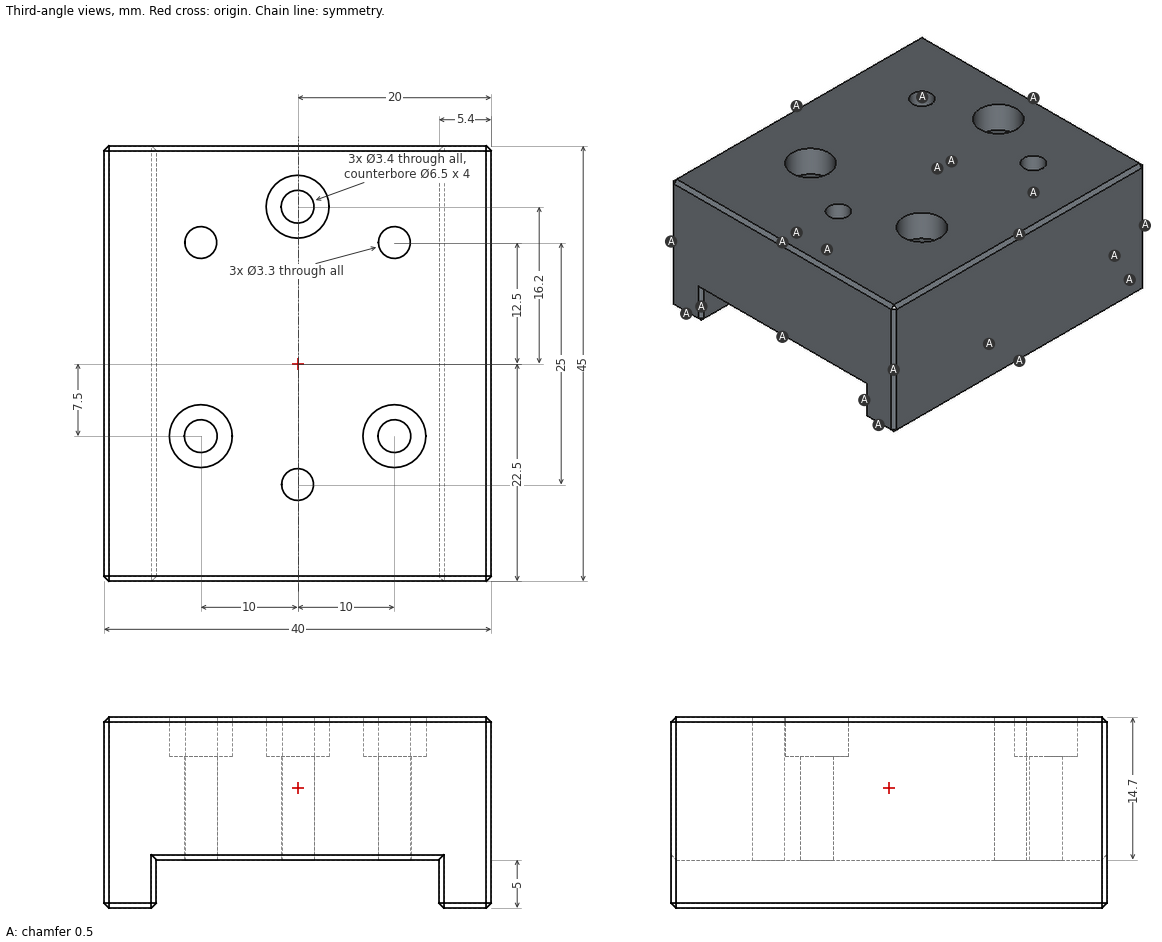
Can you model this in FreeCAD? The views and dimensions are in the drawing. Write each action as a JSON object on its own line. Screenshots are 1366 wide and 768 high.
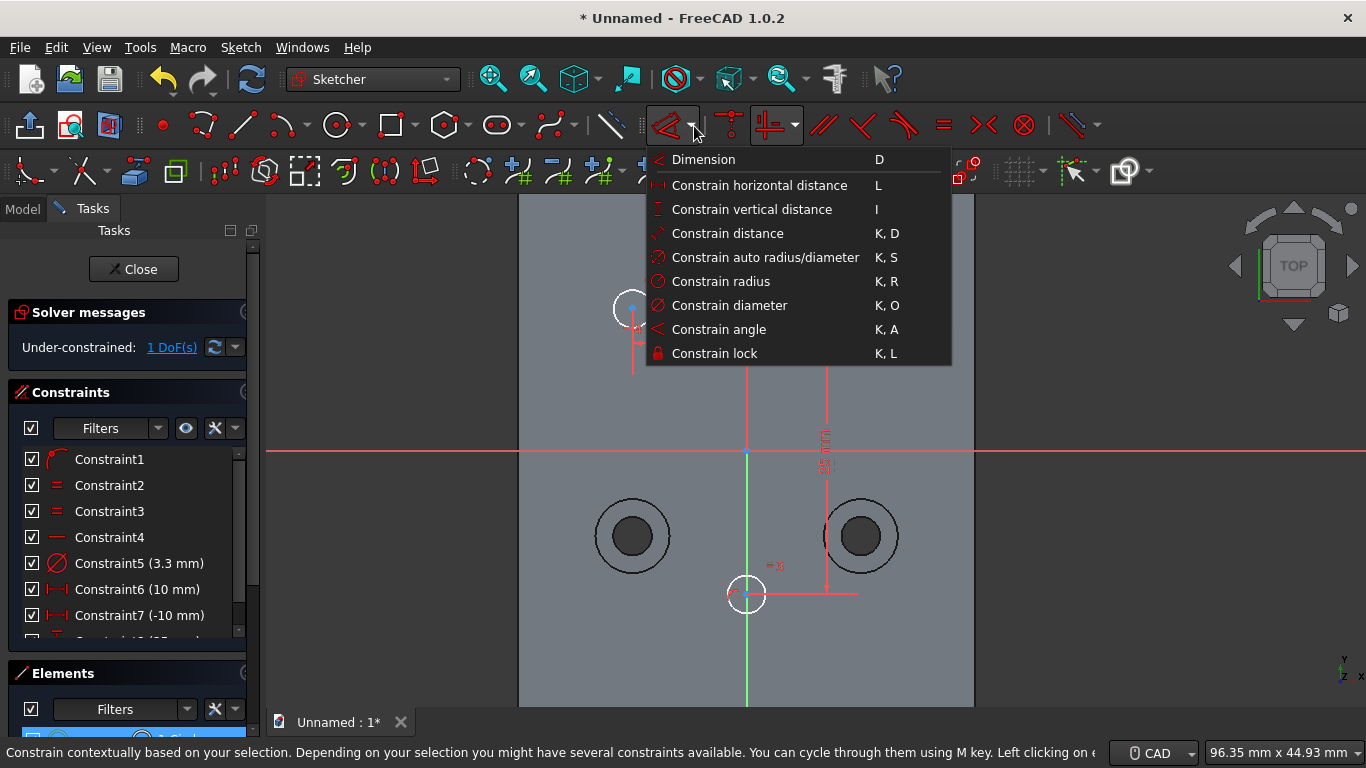
{"action": "left_click", "coordinate": [799, 209]}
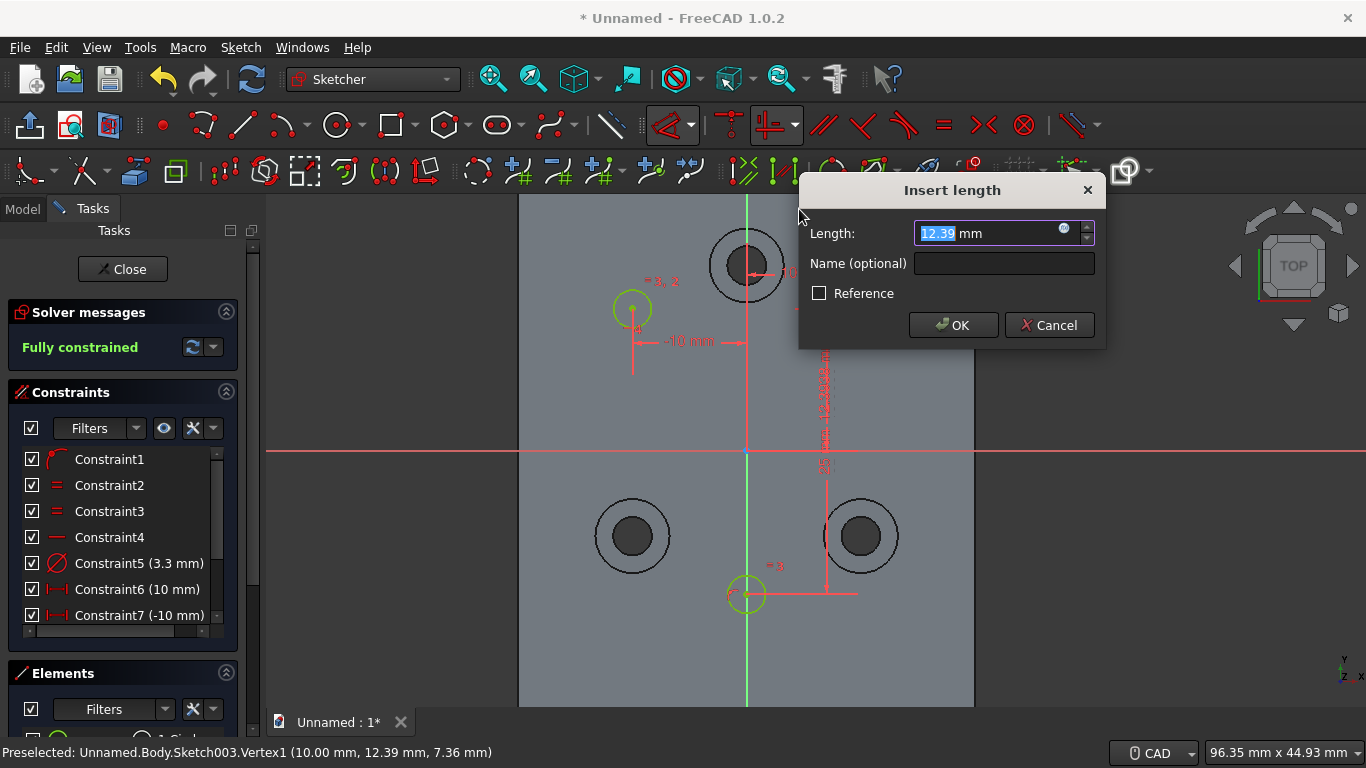
{"action": "type", "text": "12.5"}
{"action": "key", "text": "Return"}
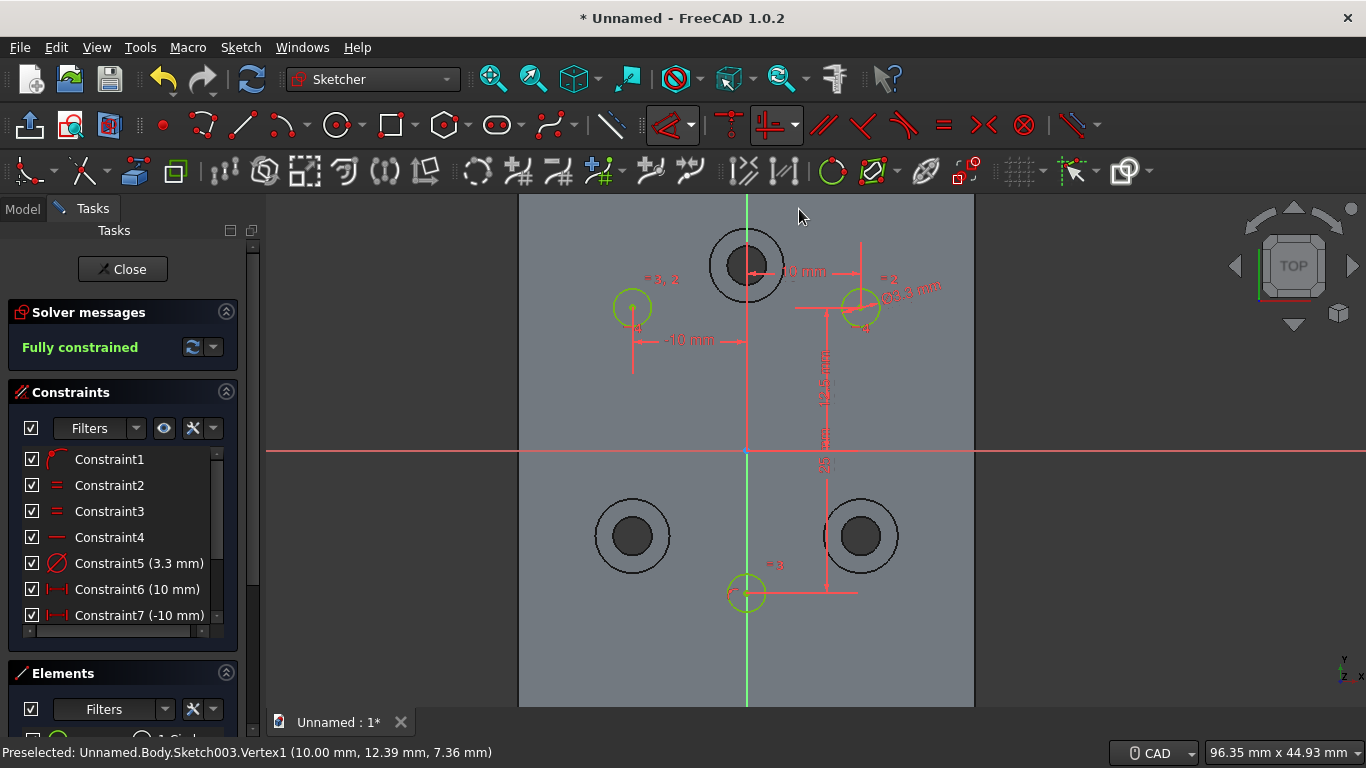
{"action": "left_click", "coordinate": [123, 269]}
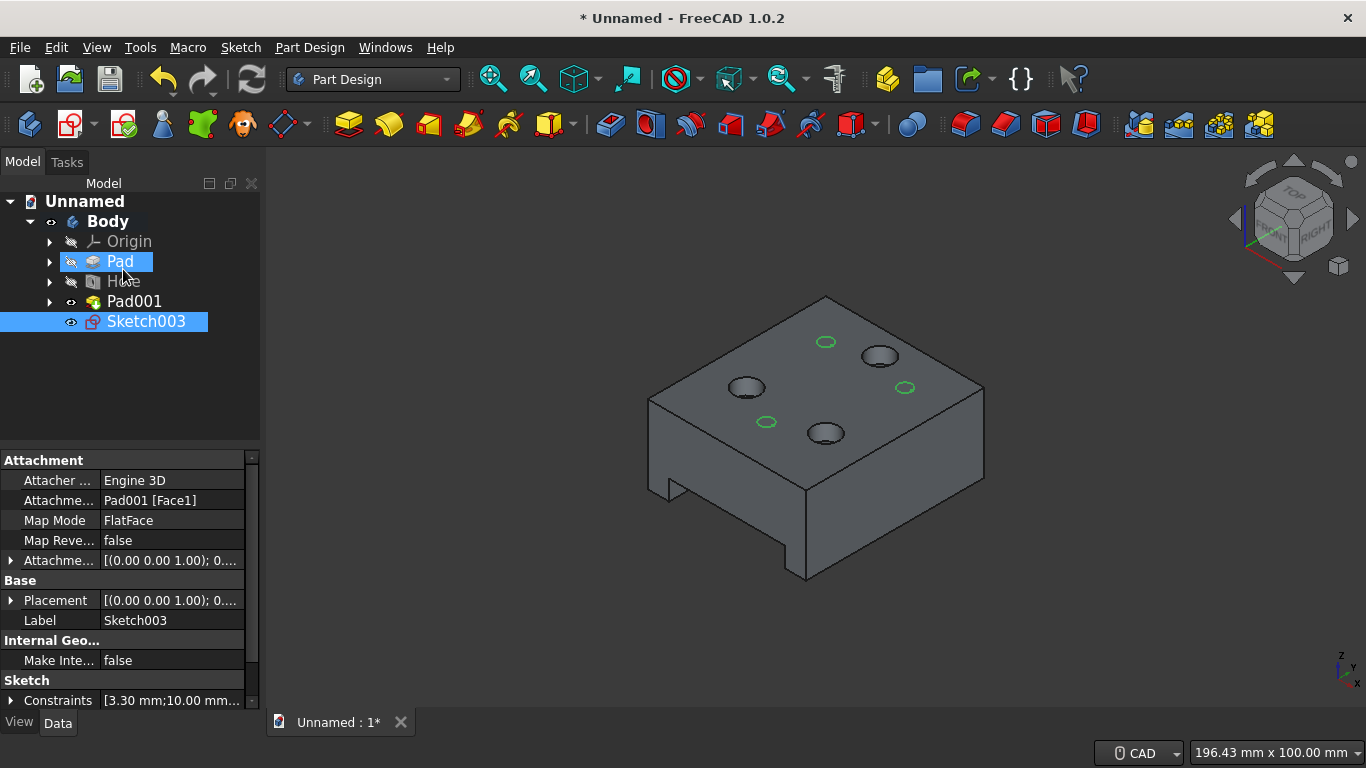
{"action": "left_click", "coordinate": [652, 124]}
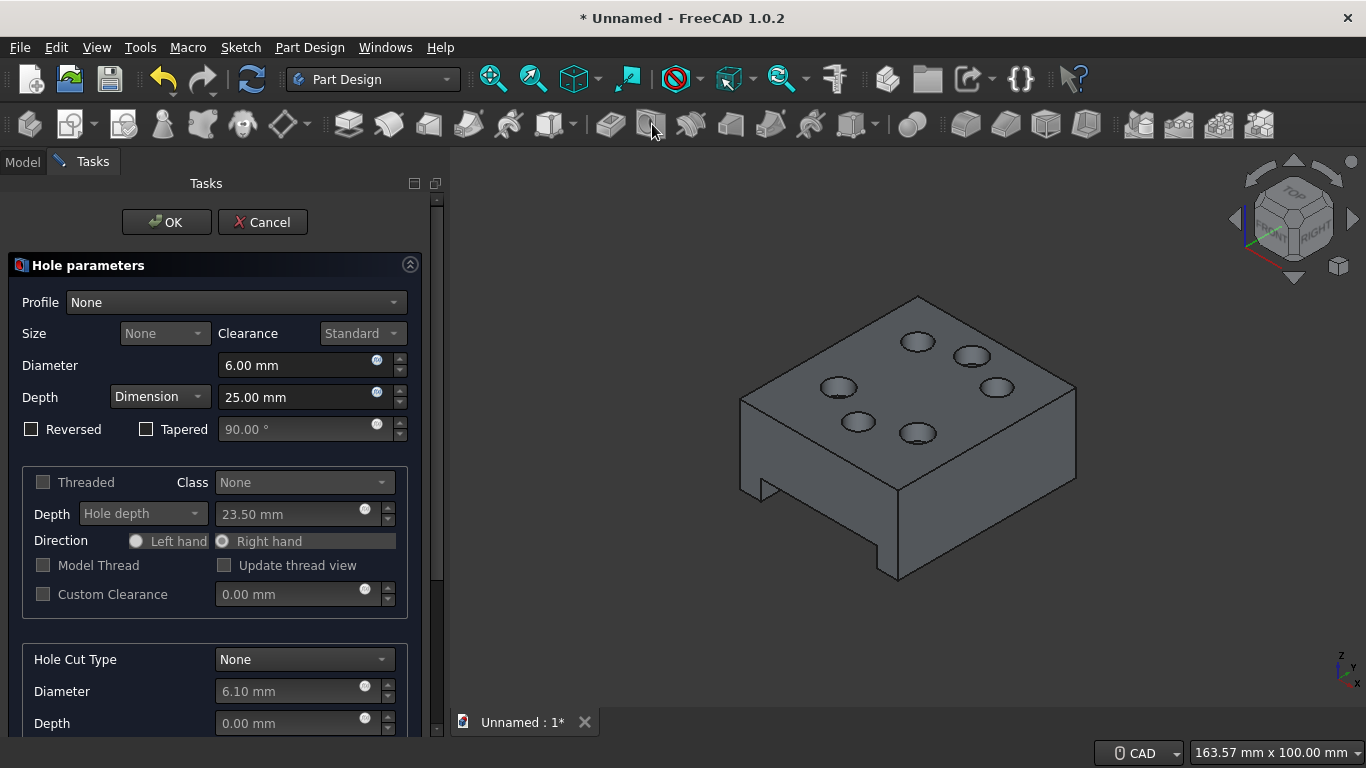
{"action": "triple_click", "coordinate": [305, 365]}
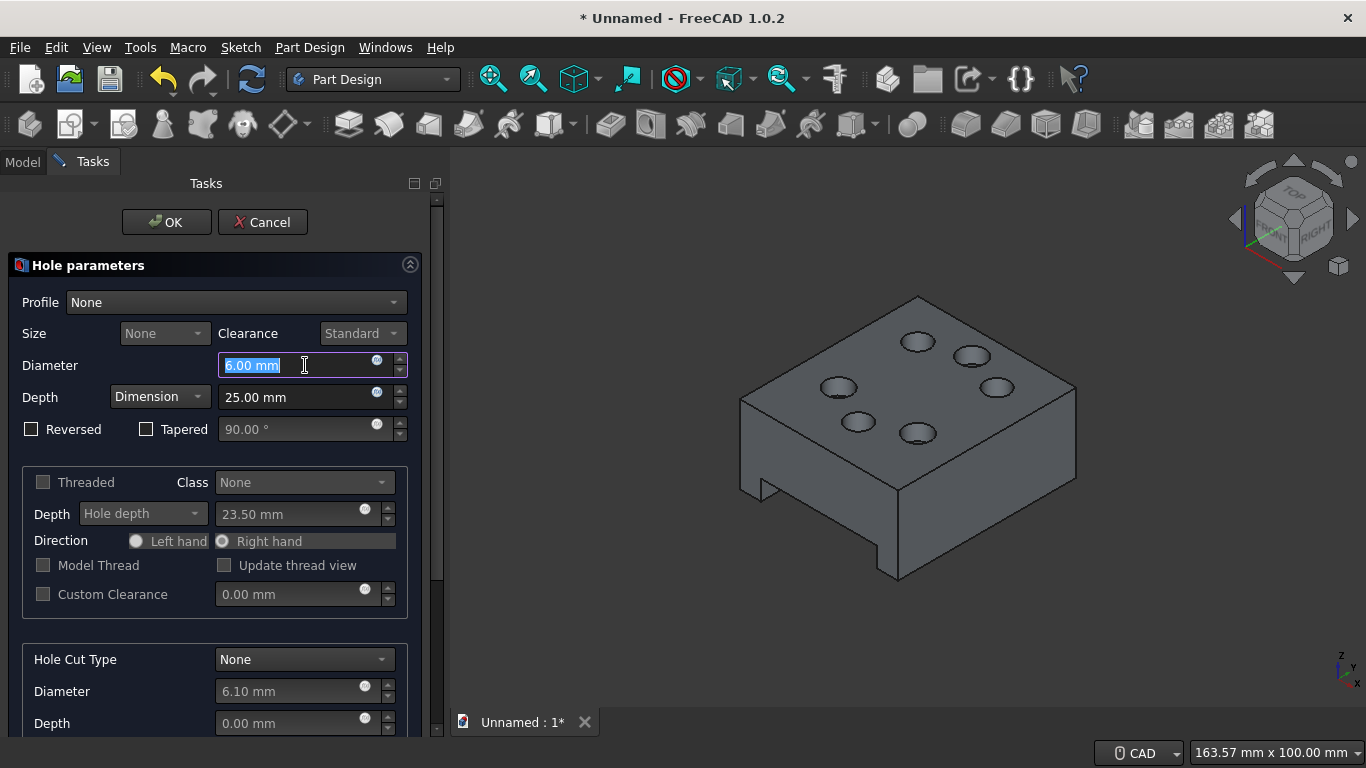
{"action": "type", "text": "3.3"}
{"action": "key", "text": "Tab"}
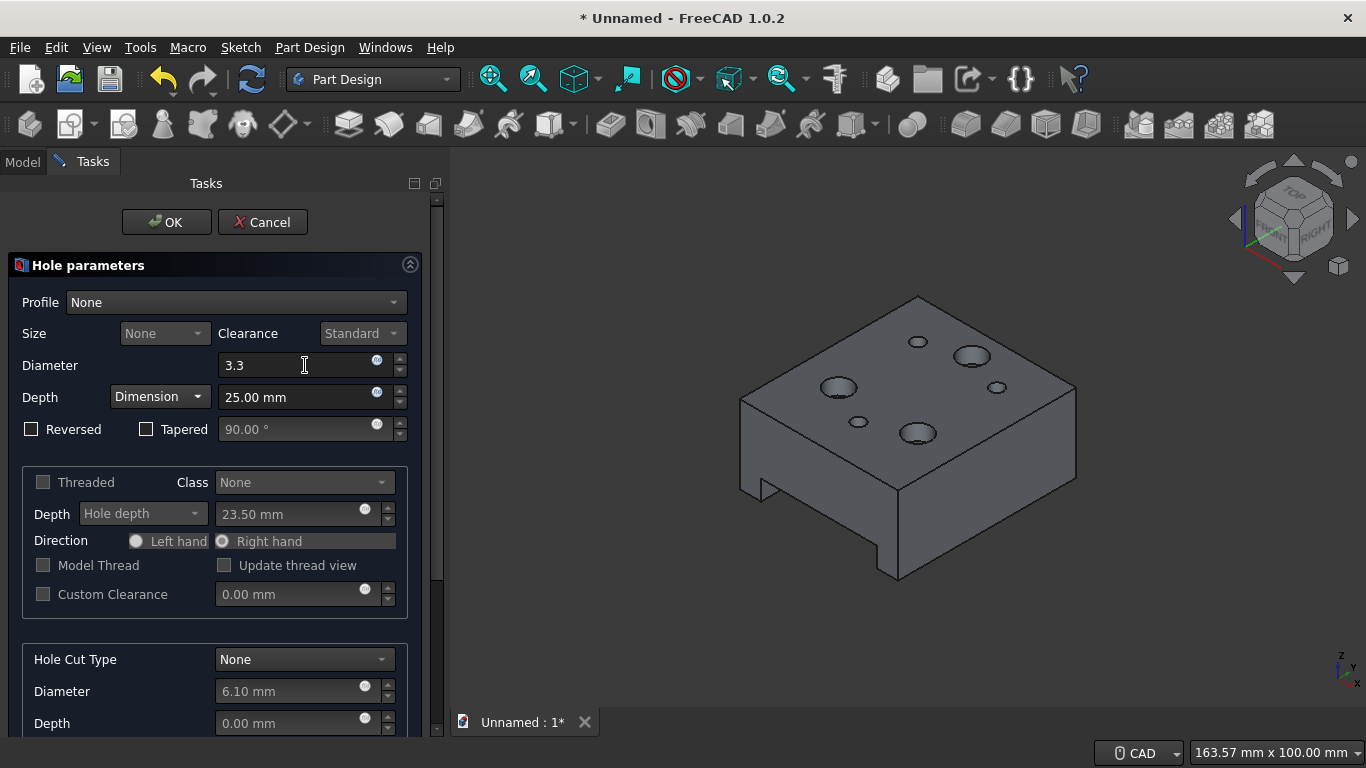
{"action": "left_click", "coordinate": [161, 396]}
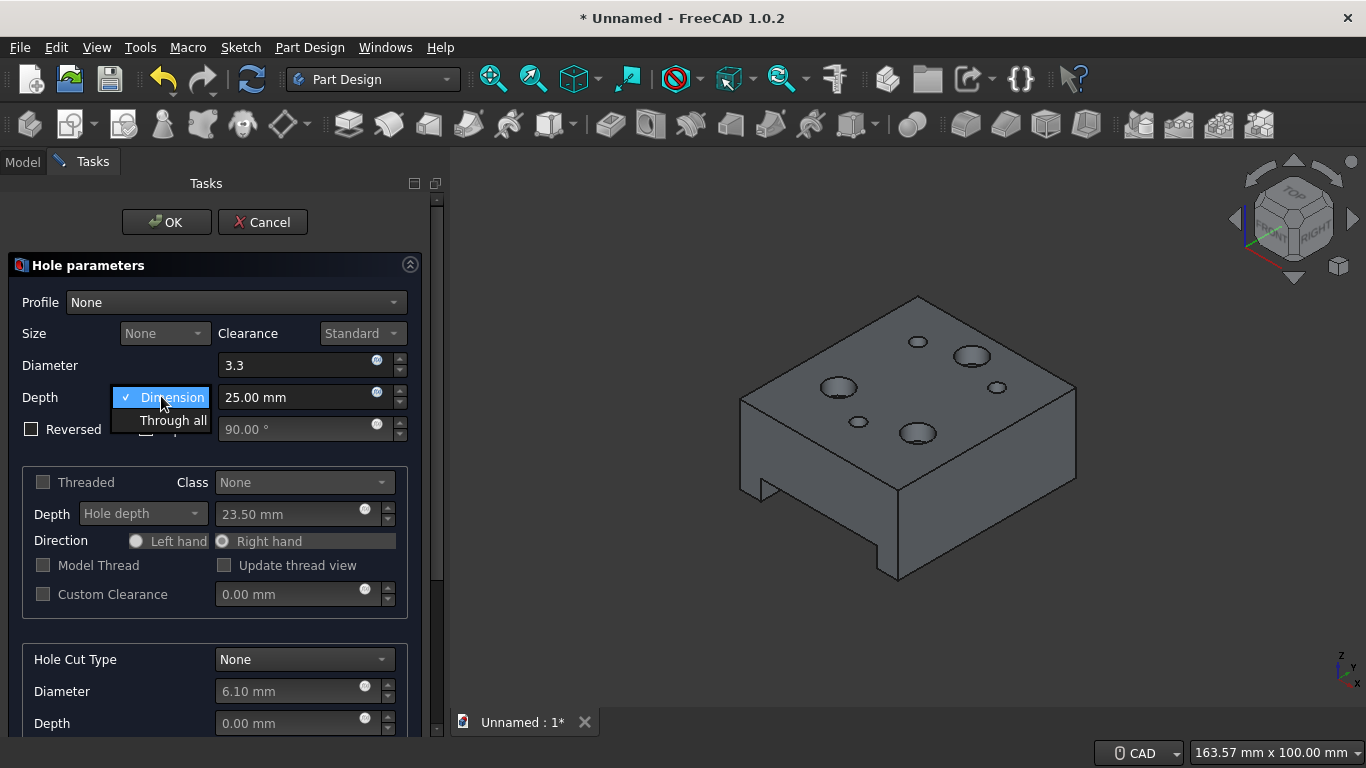
{"action": "left_click", "coordinate": [160, 420]}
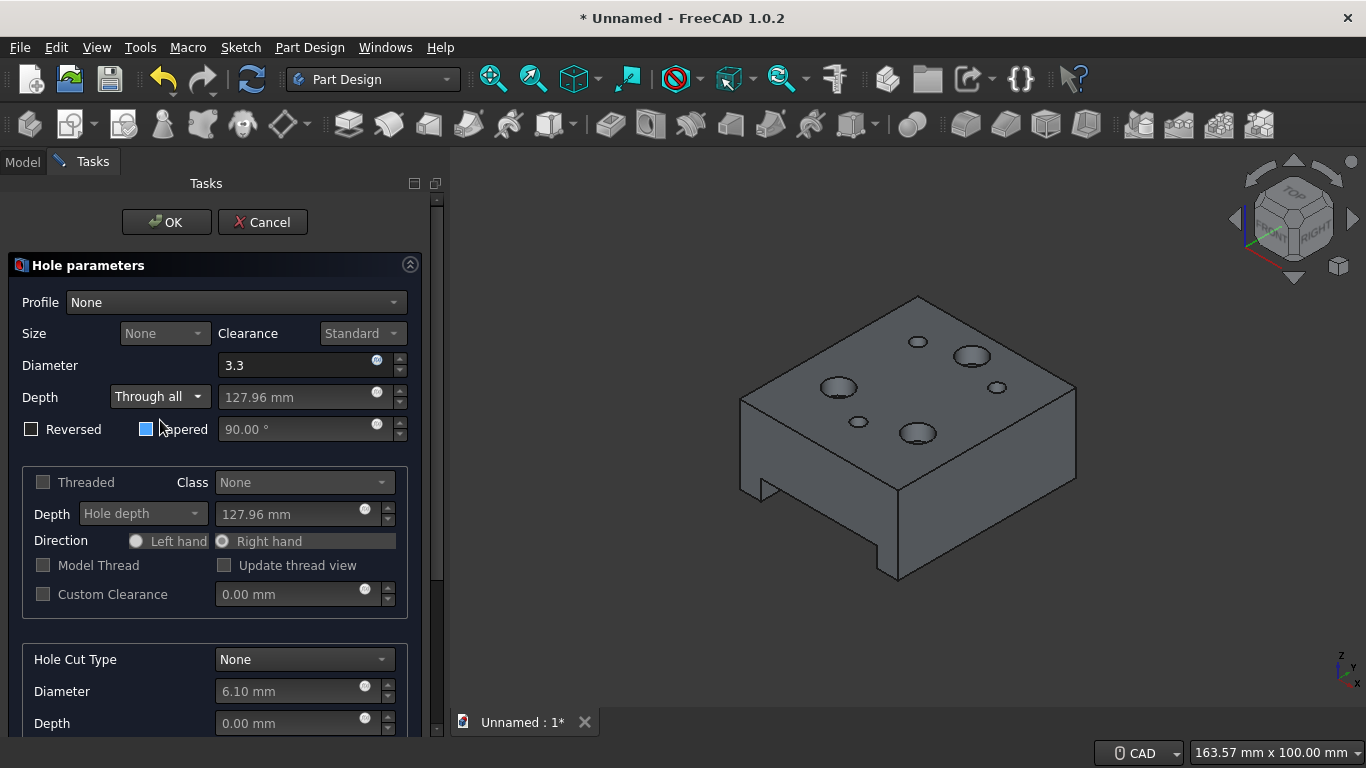
{"action": "left_click", "coordinate": [167, 222]}